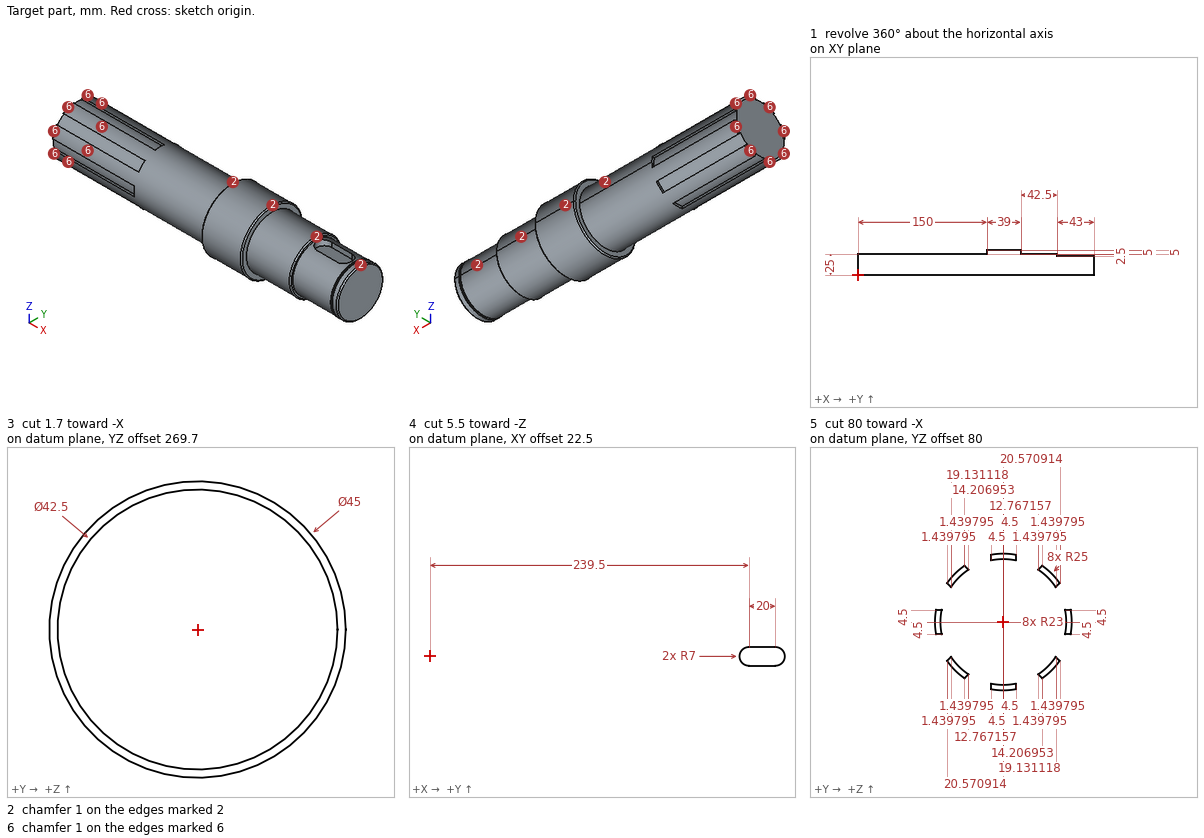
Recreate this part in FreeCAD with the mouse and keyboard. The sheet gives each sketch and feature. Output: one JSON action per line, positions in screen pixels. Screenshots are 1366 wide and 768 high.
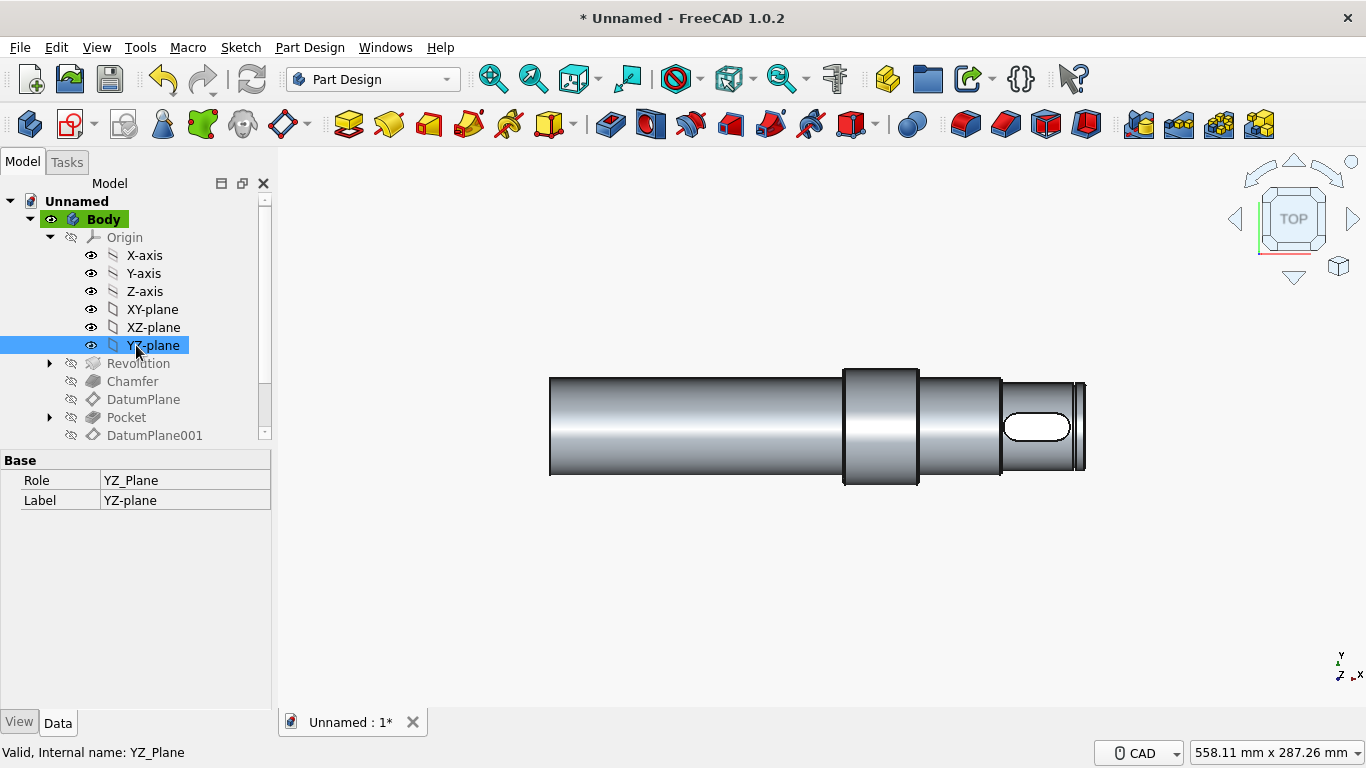
{"action": "left_click", "coordinate": [284, 124]}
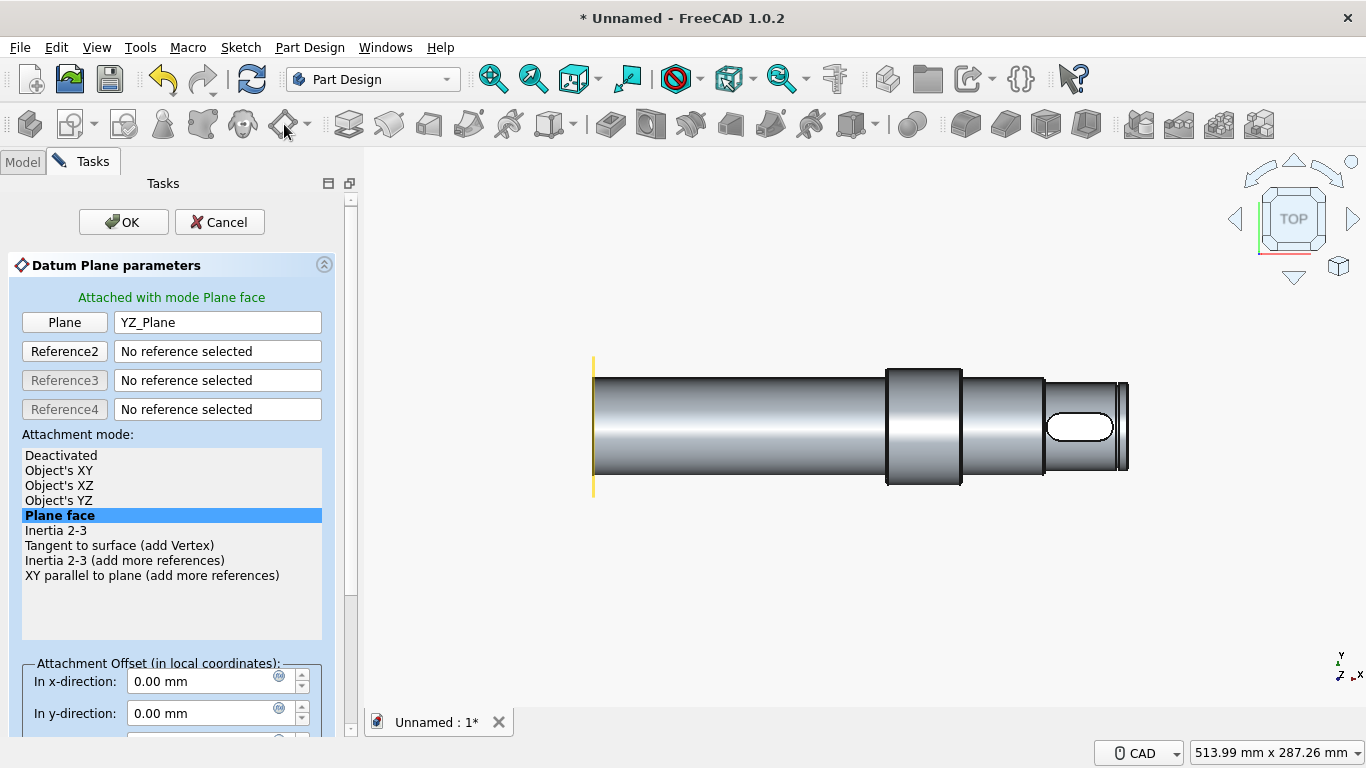
{"action": "scroll", "coordinate": [351, 464], "scroll_direction": "down", "scroll_amount": 2}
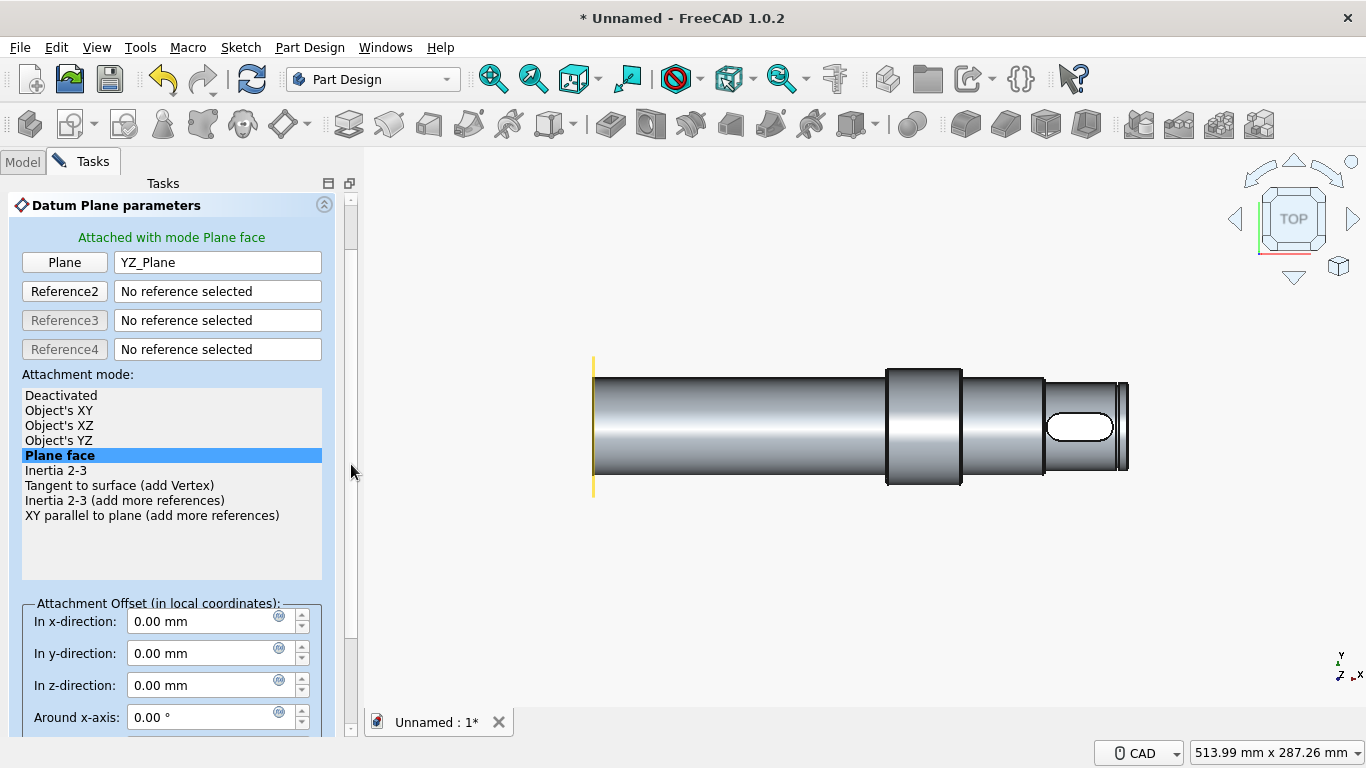
{"action": "triple_click", "coordinate": [210, 625]}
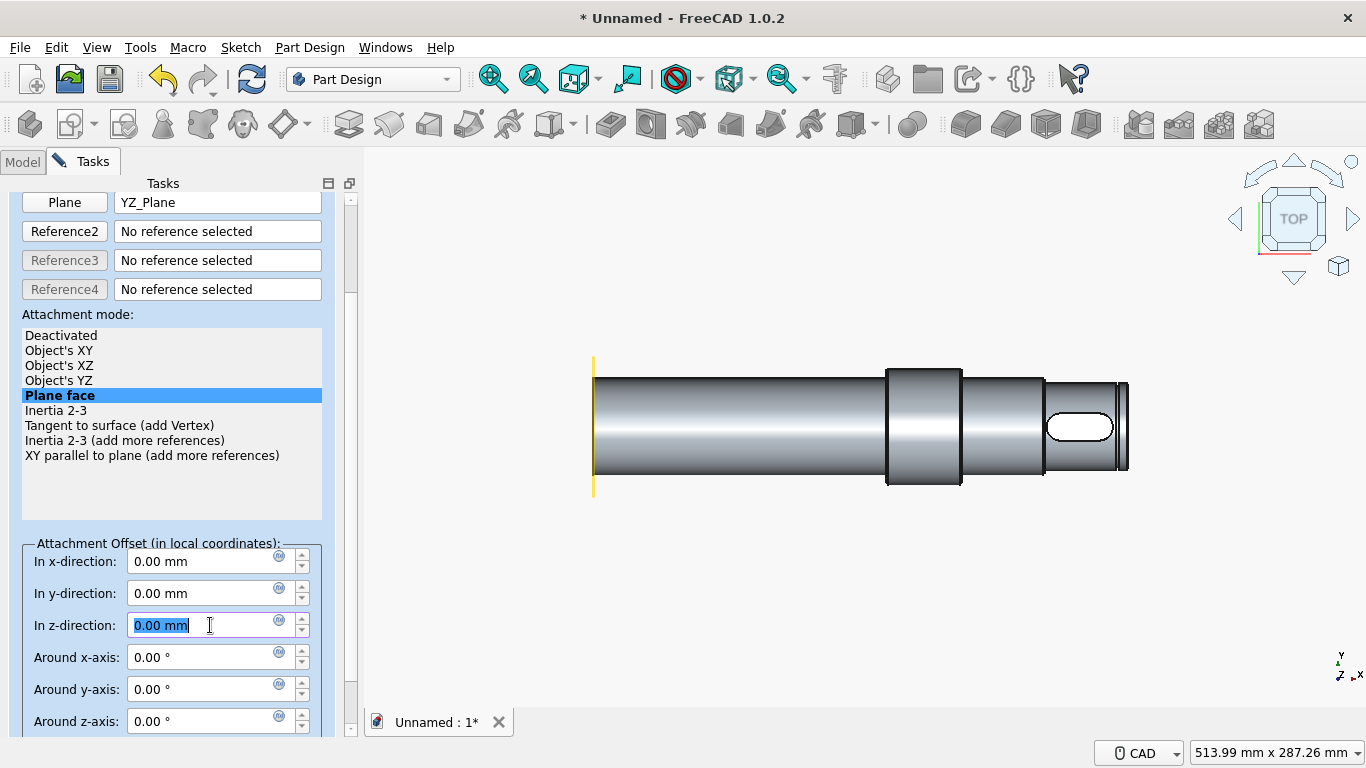
{"action": "type", "text": "80"}
{"action": "key", "text": "Tab"}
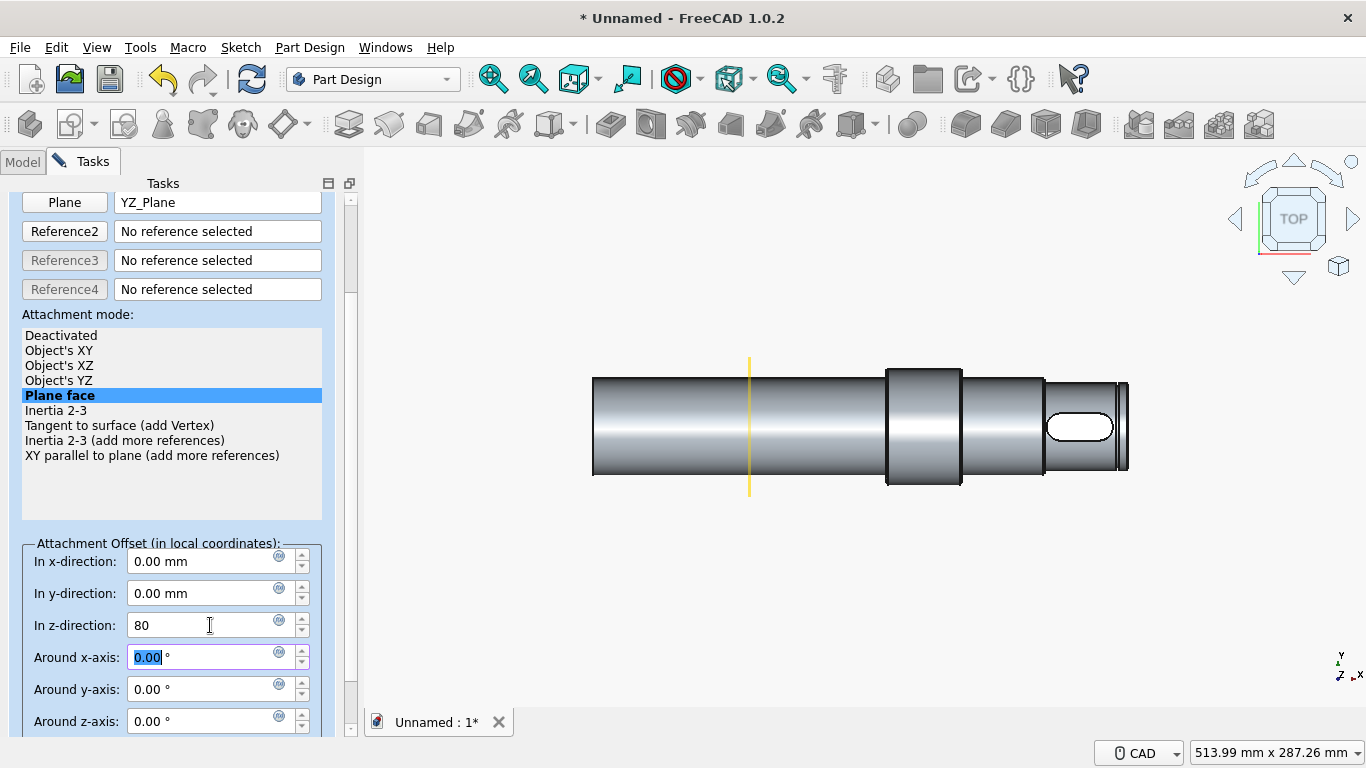
{"action": "scroll", "coordinate": [351, 464], "scroll_direction": "up", "scroll_amount": 3}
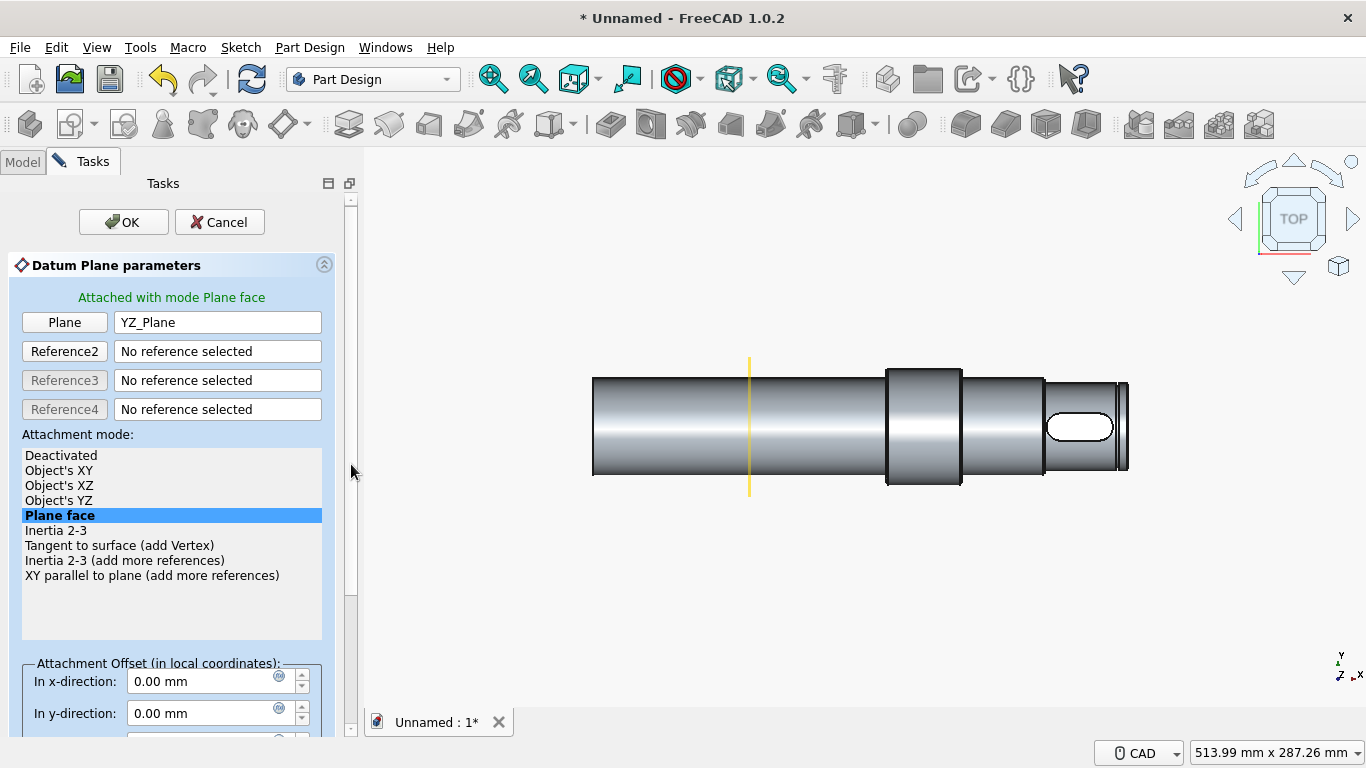
{"action": "left_click", "coordinate": [124, 222]}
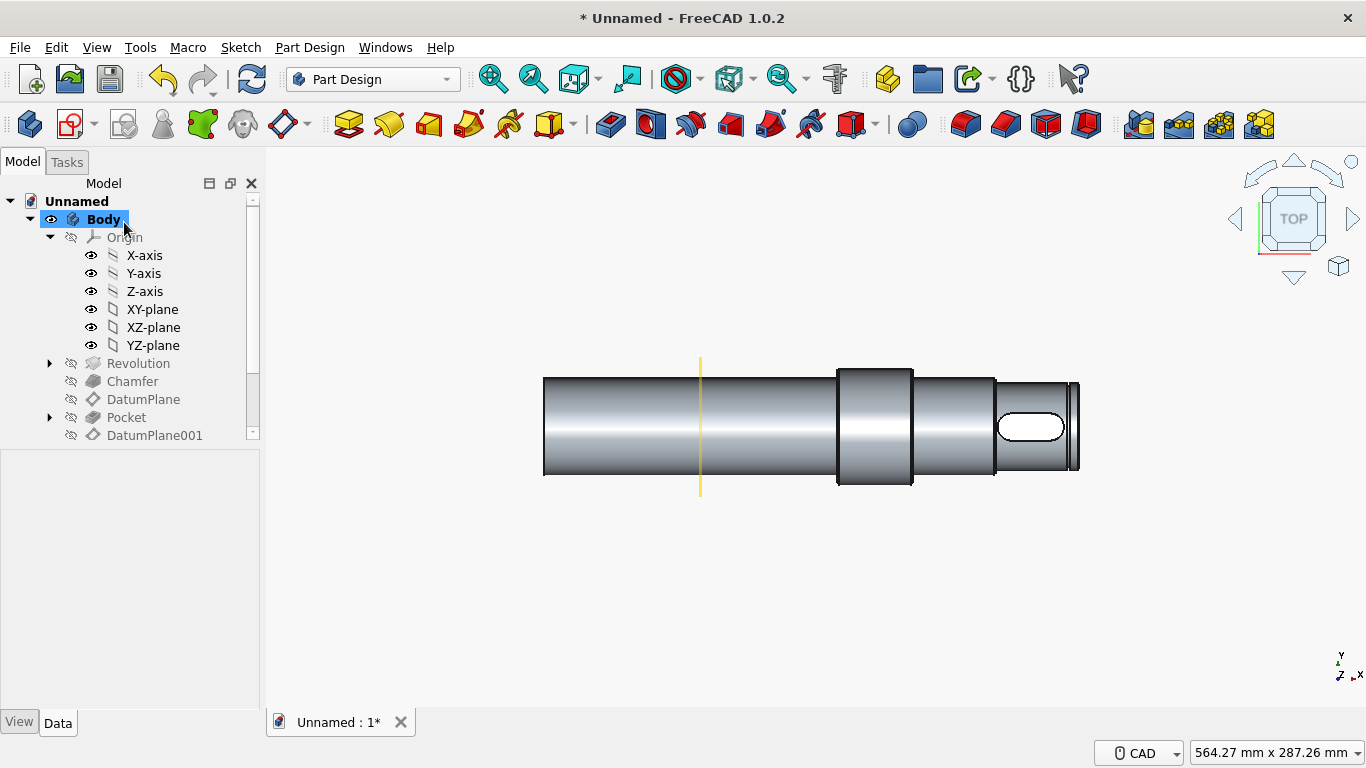
{"action": "scroll", "coordinate": [100, 323], "scroll_direction": "down", "scroll_amount": 3}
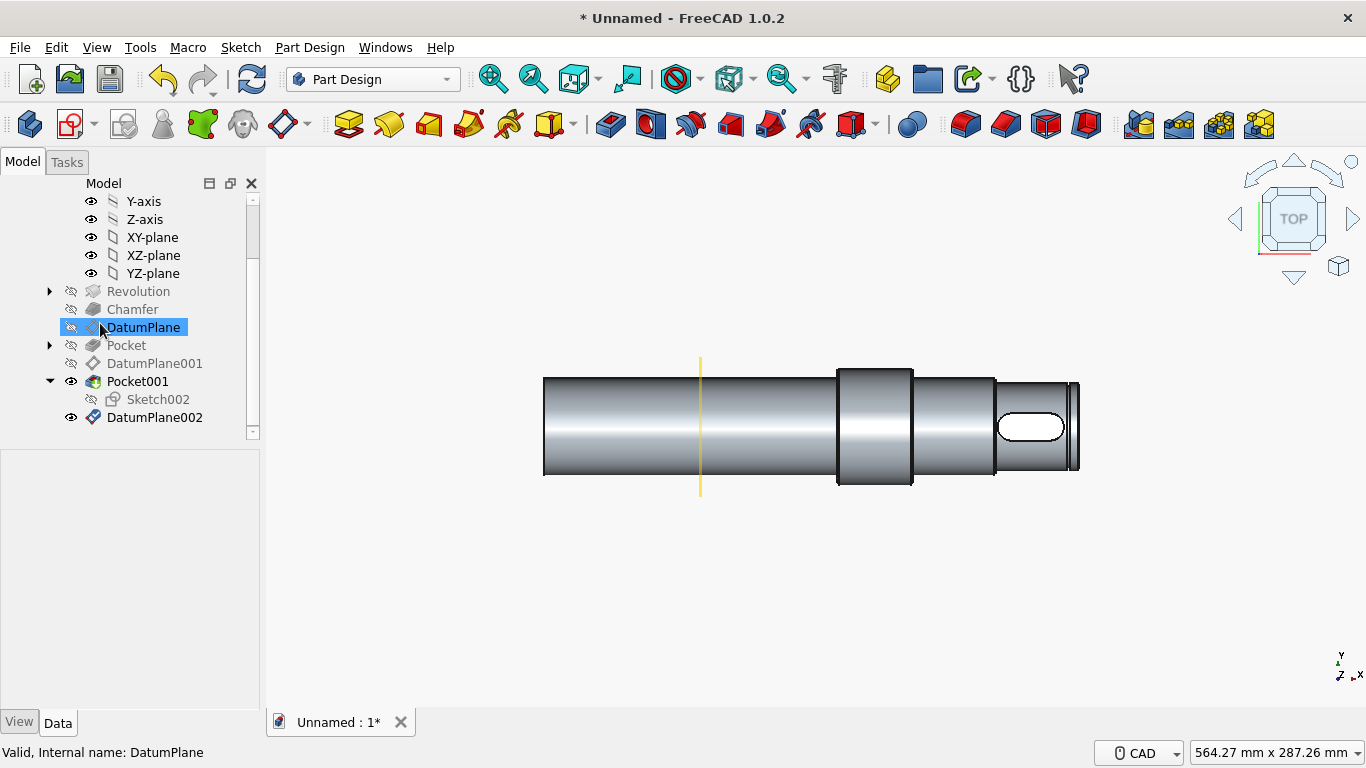
{"action": "left_click", "coordinate": [116, 417]}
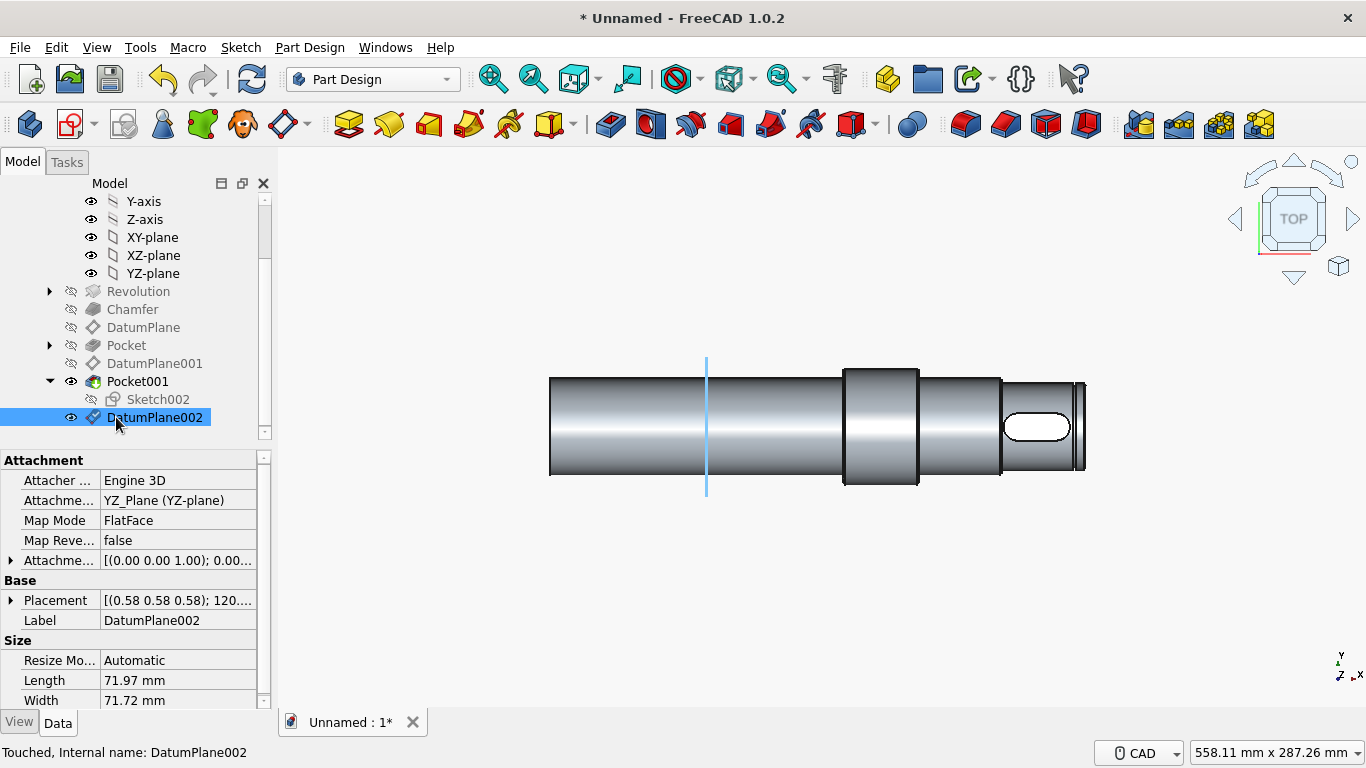
{"action": "left_click", "coordinate": [70, 124]}